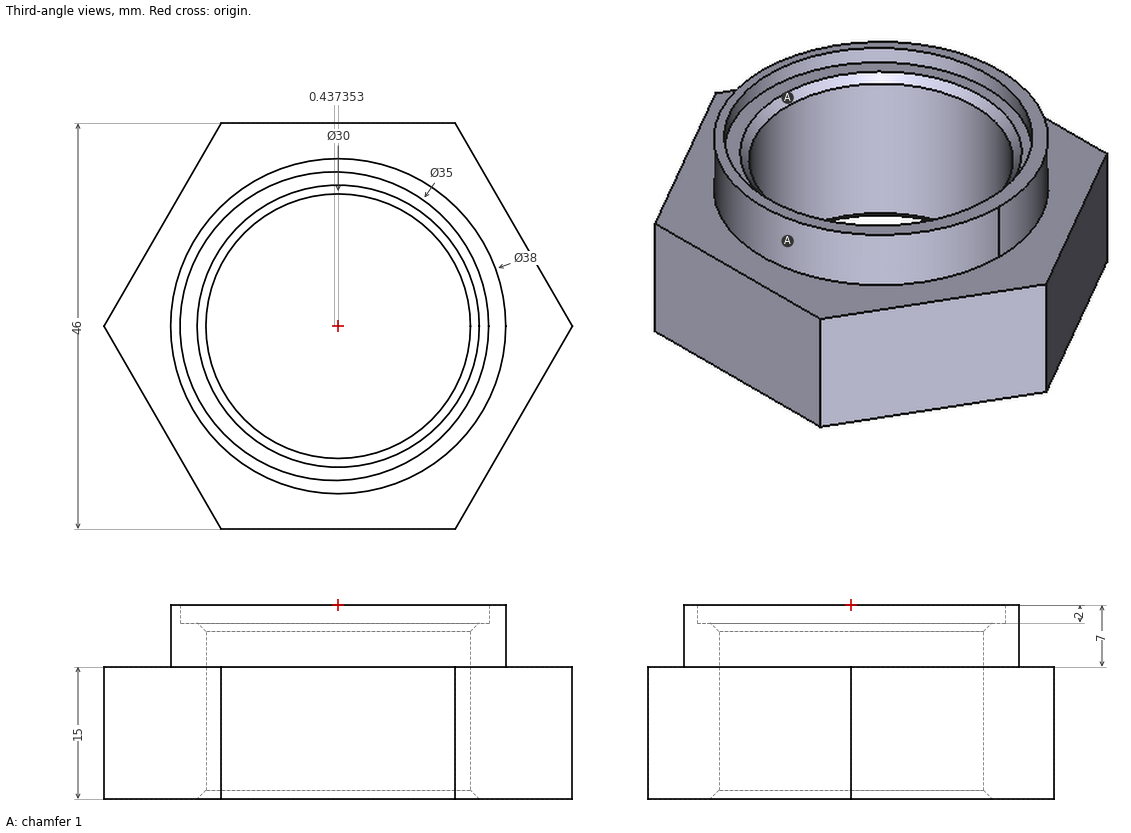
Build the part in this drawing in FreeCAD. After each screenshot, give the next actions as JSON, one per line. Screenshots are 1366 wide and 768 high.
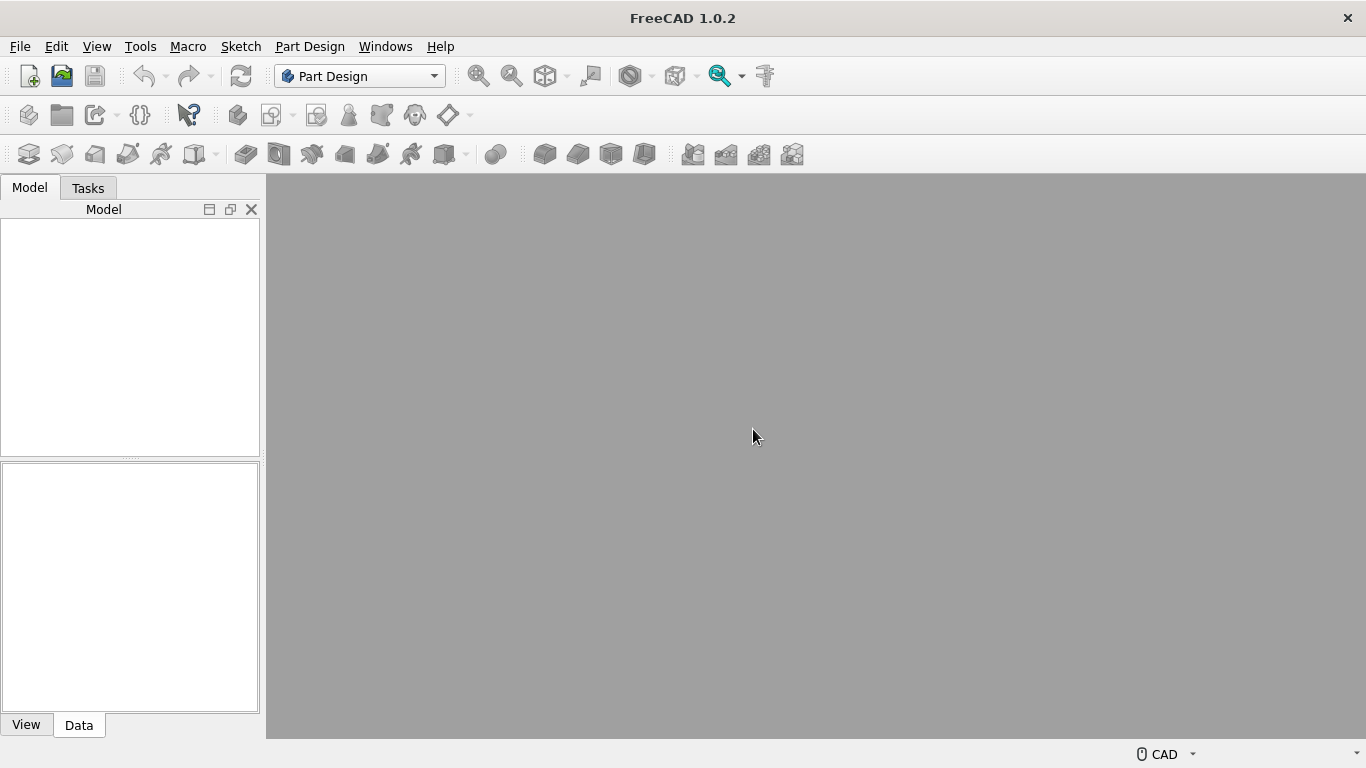
{"action": "left_click", "coordinate": [29, 76]}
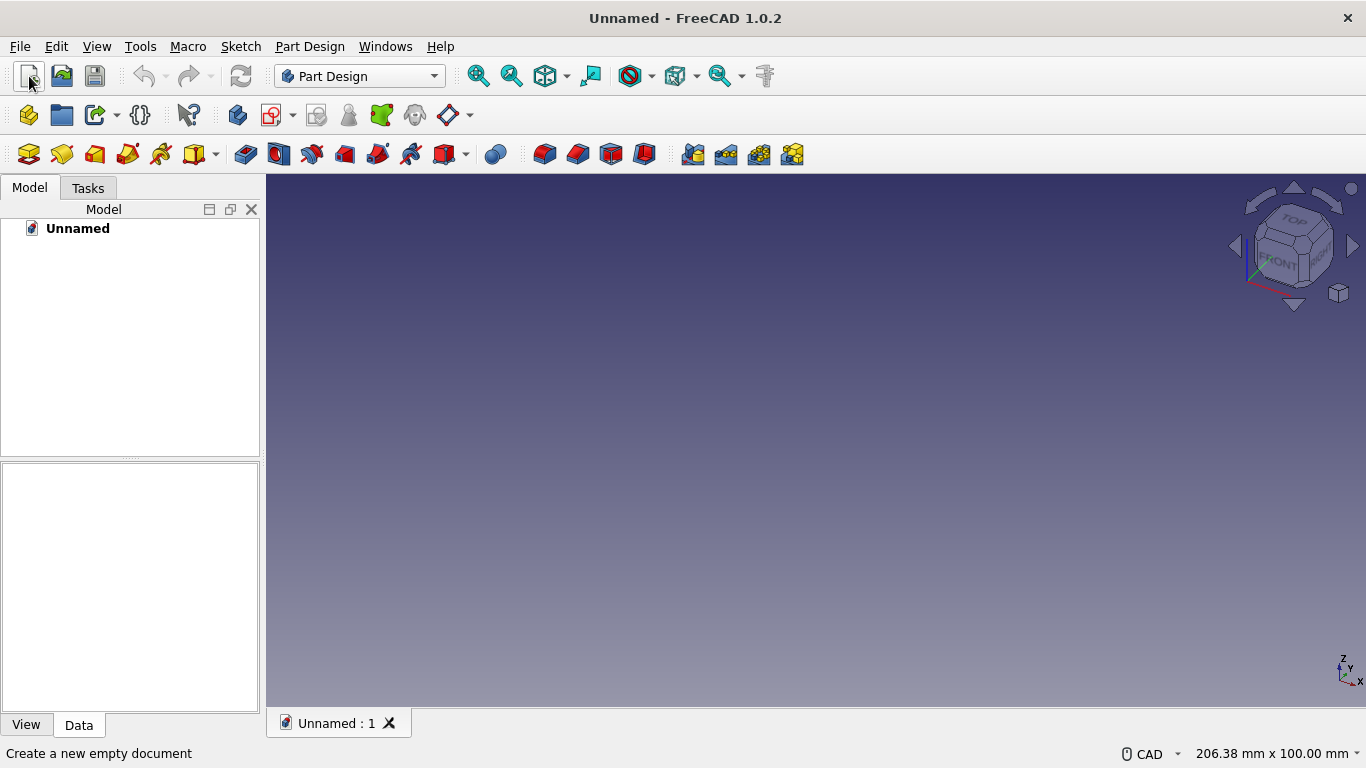
{"action": "left_click", "coordinate": [270, 116]}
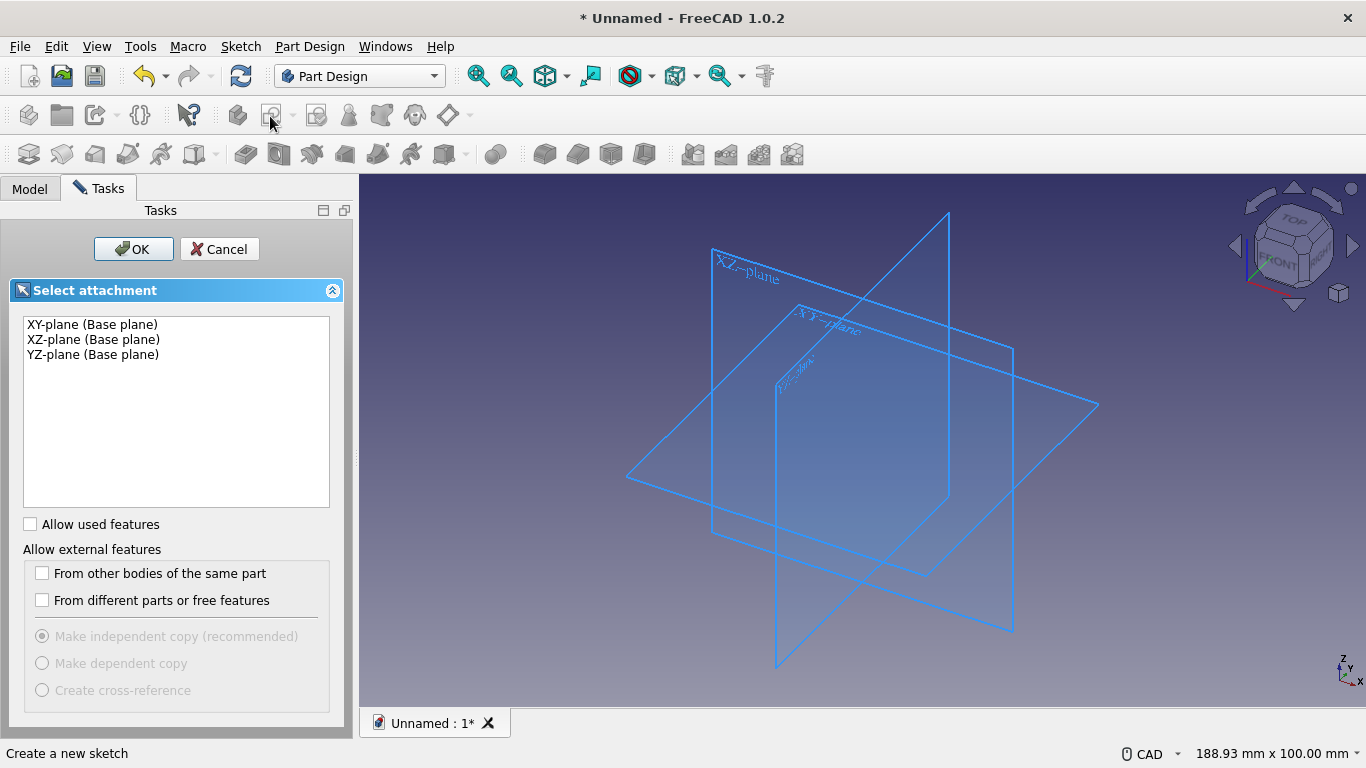
{"action": "left_click", "coordinate": [84, 324]}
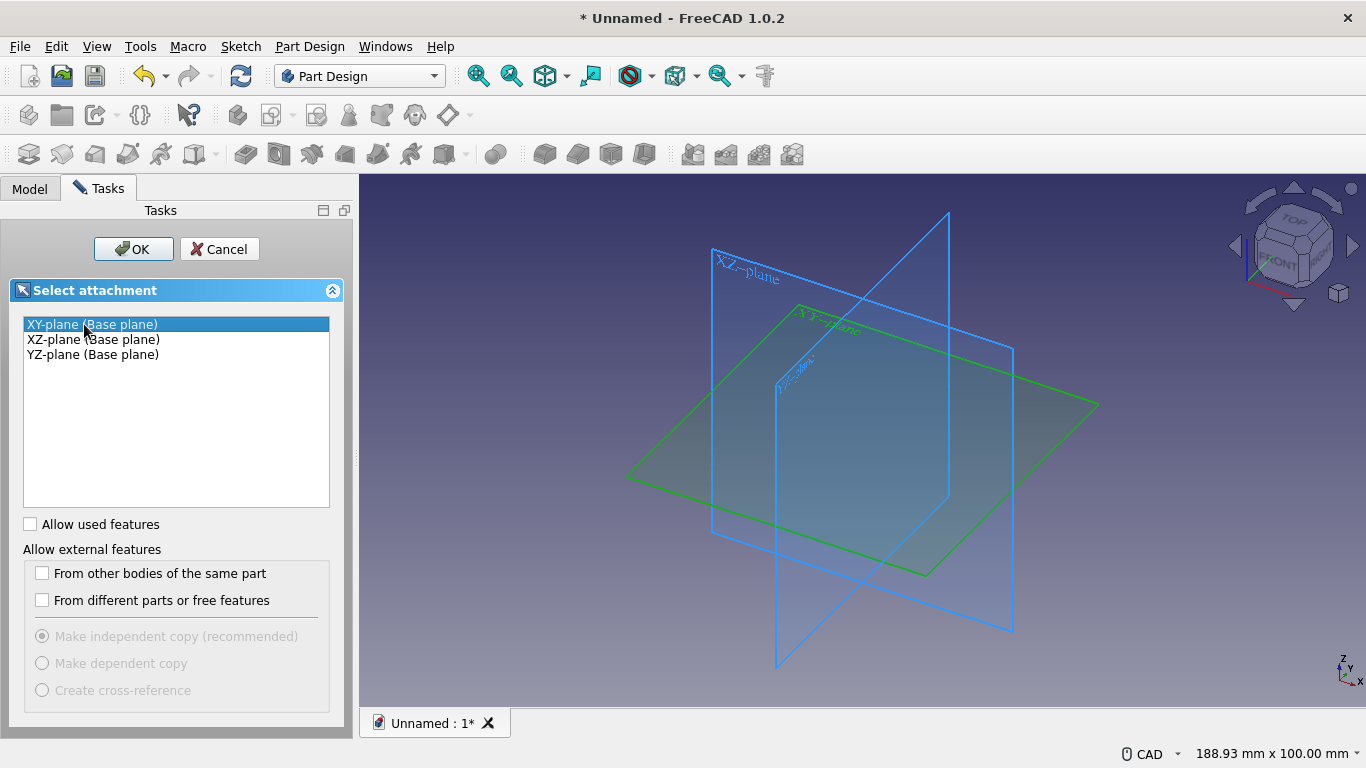
{"action": "left_click", "coordinate": [134, 249]}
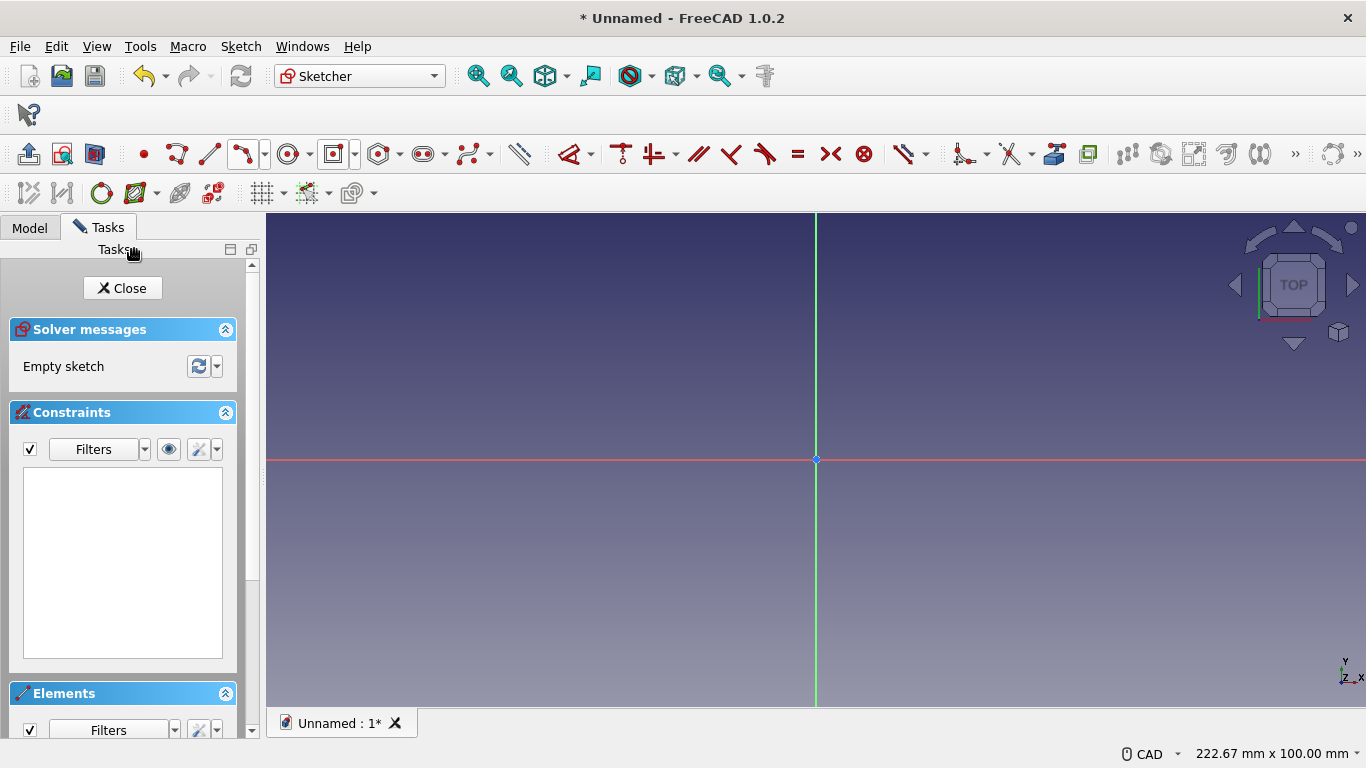
{"action": "scroll", "coordinate": [955, 460], "scroll_direction": "up", "scroll_amount": 2}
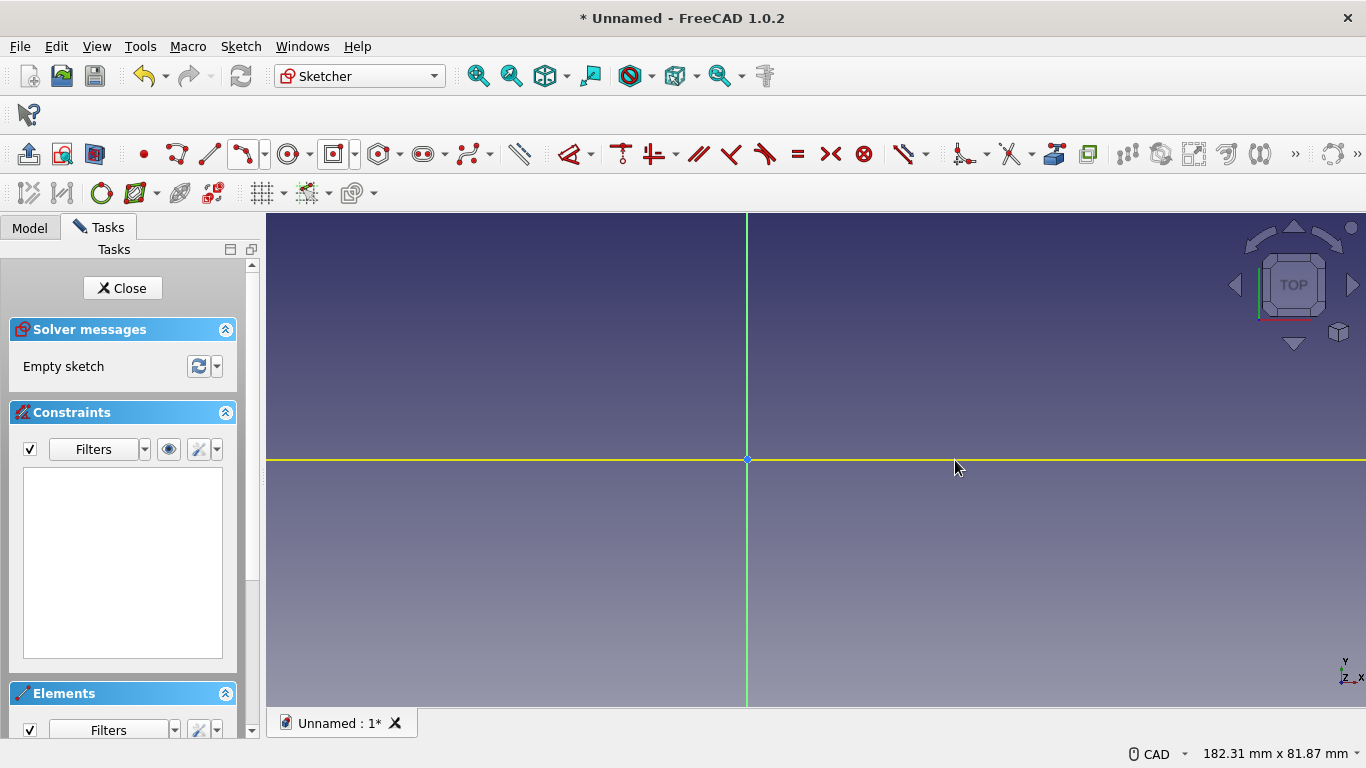
{"action": "left_click", "coordinate": [288, 154]}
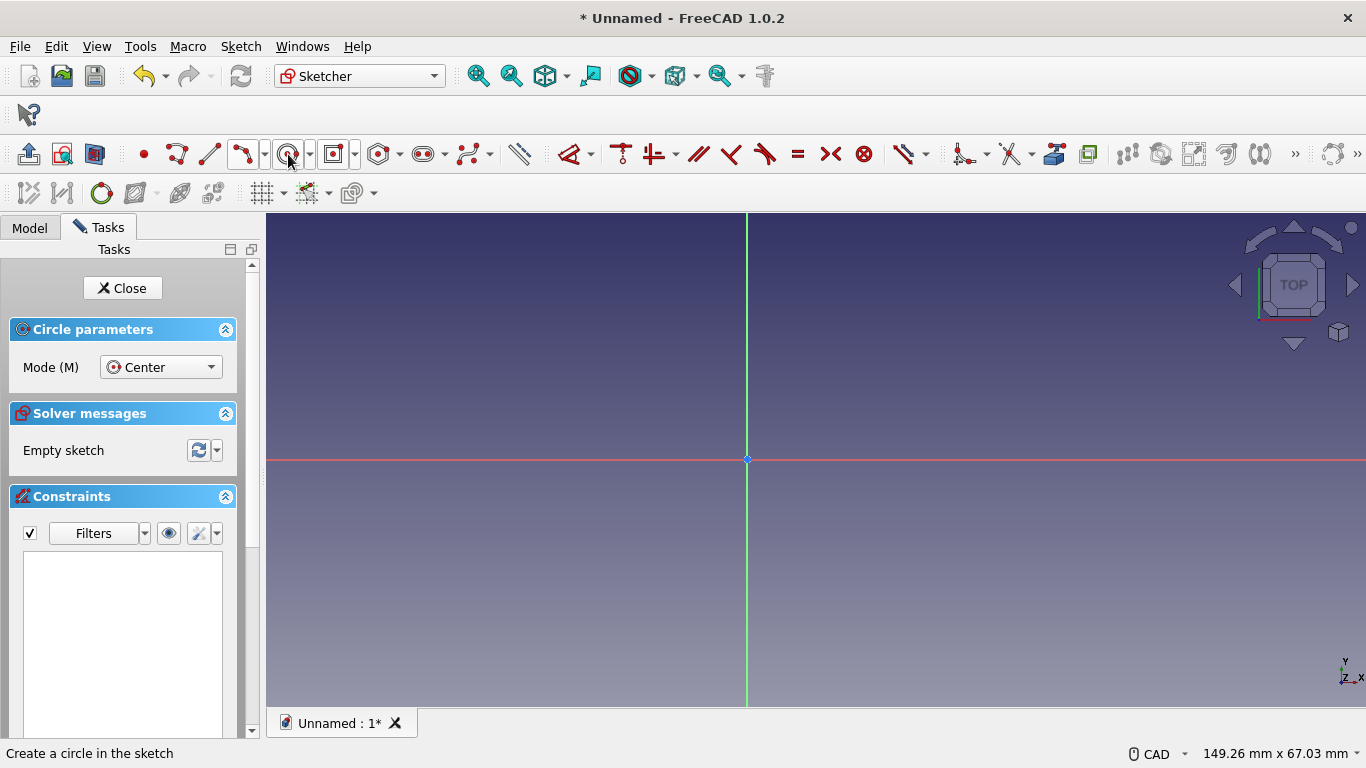
{"action": "left_click", "coordinate": [747, 460]}
{"action": "mouse_move", "coordinate": [846, 361]}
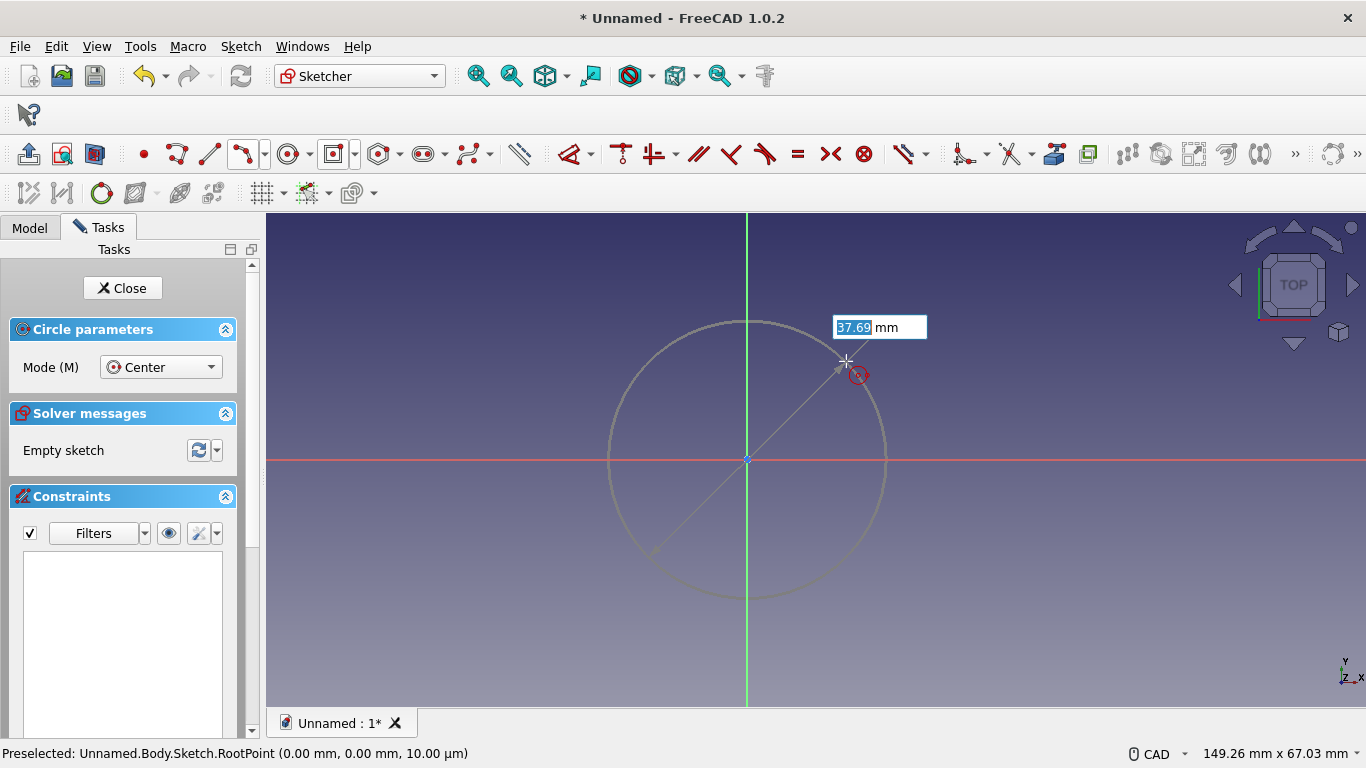
{"action": "type", "text": "38"}
{"action": "key", "text": "Return"}
{"action": "key", "text": "Escape"}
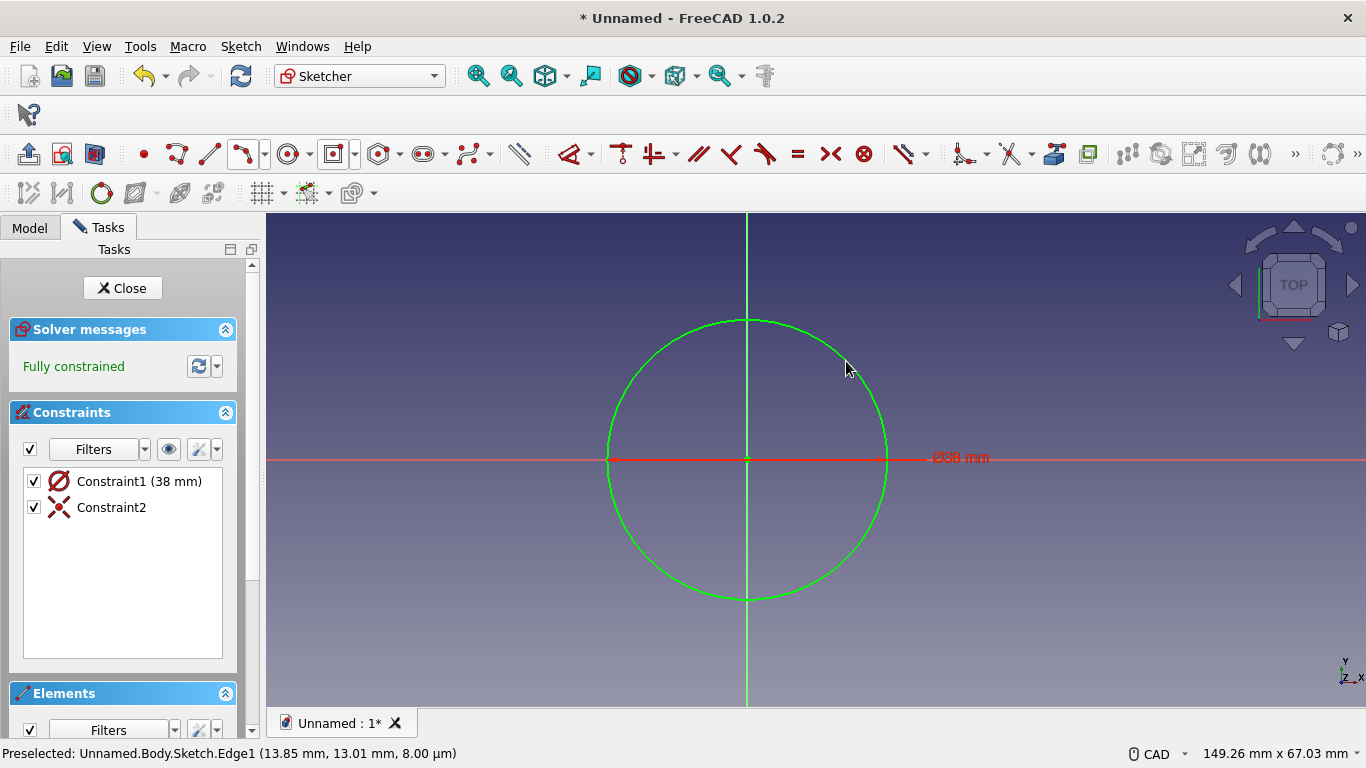
{"action": "left_click", "coordinate": [123, 288]}